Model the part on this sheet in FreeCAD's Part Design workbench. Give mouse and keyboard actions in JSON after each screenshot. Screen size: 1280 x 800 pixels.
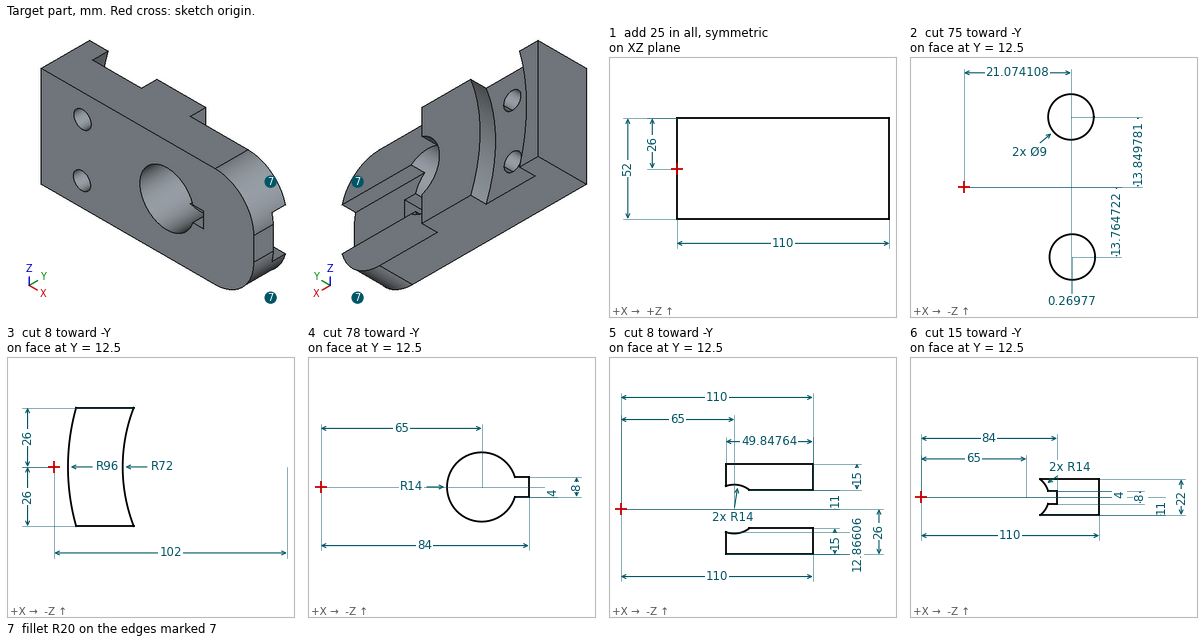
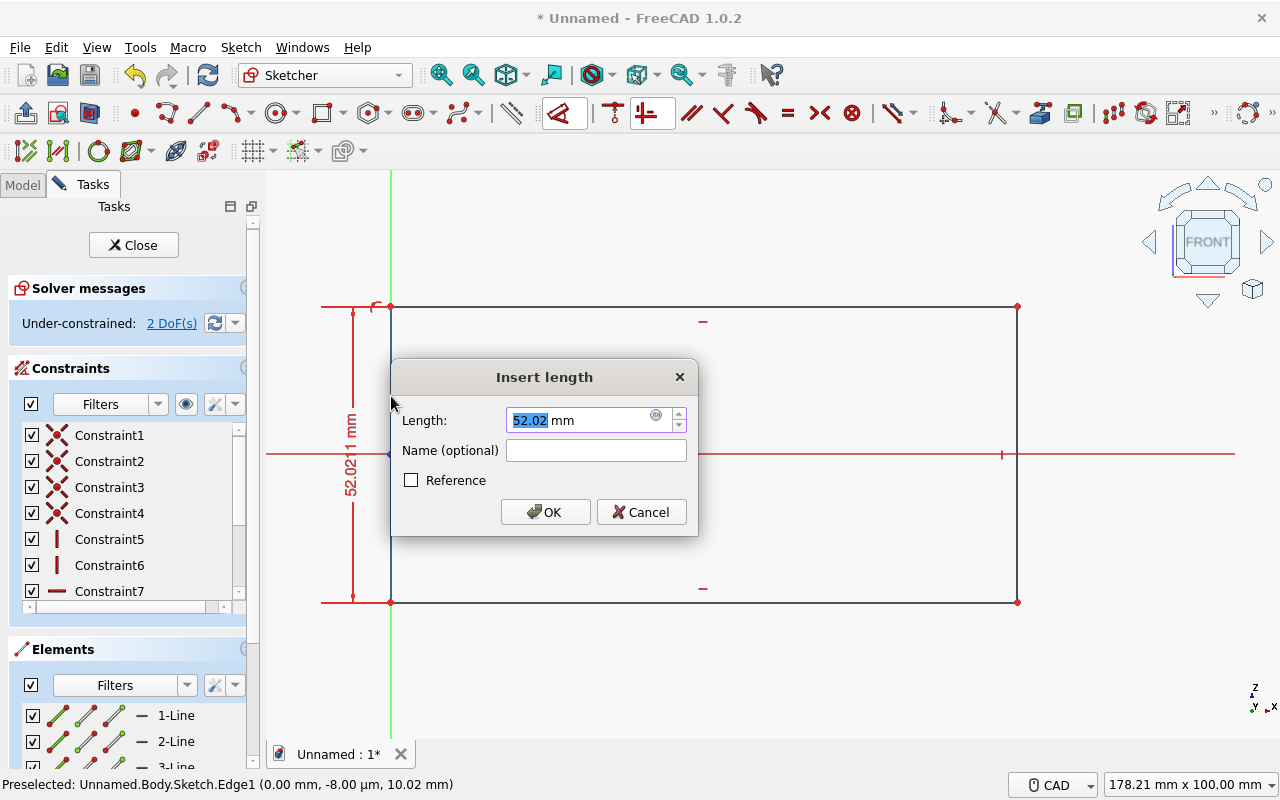
{"action": "type", "text": "52"}
{"action": "key", "text": "Return"}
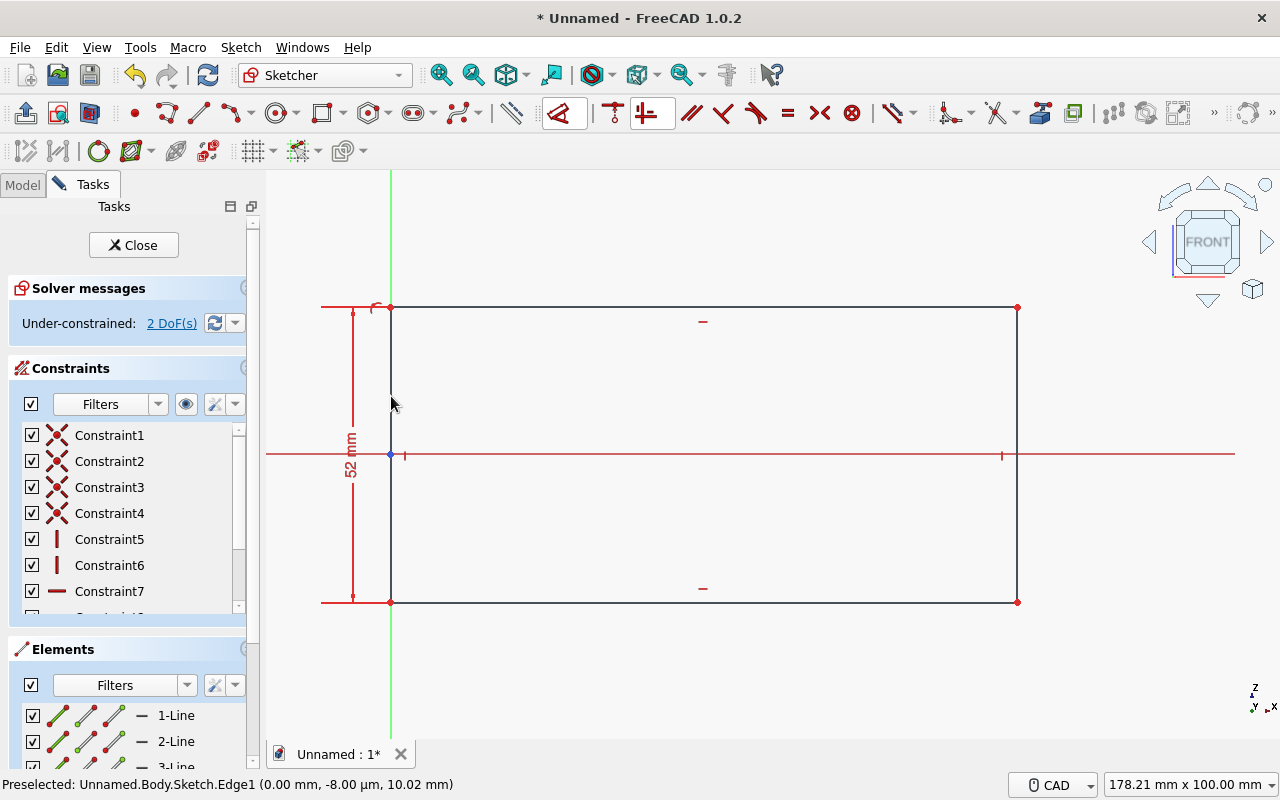
{"action": "left_click", "coordinate": [579, 603]}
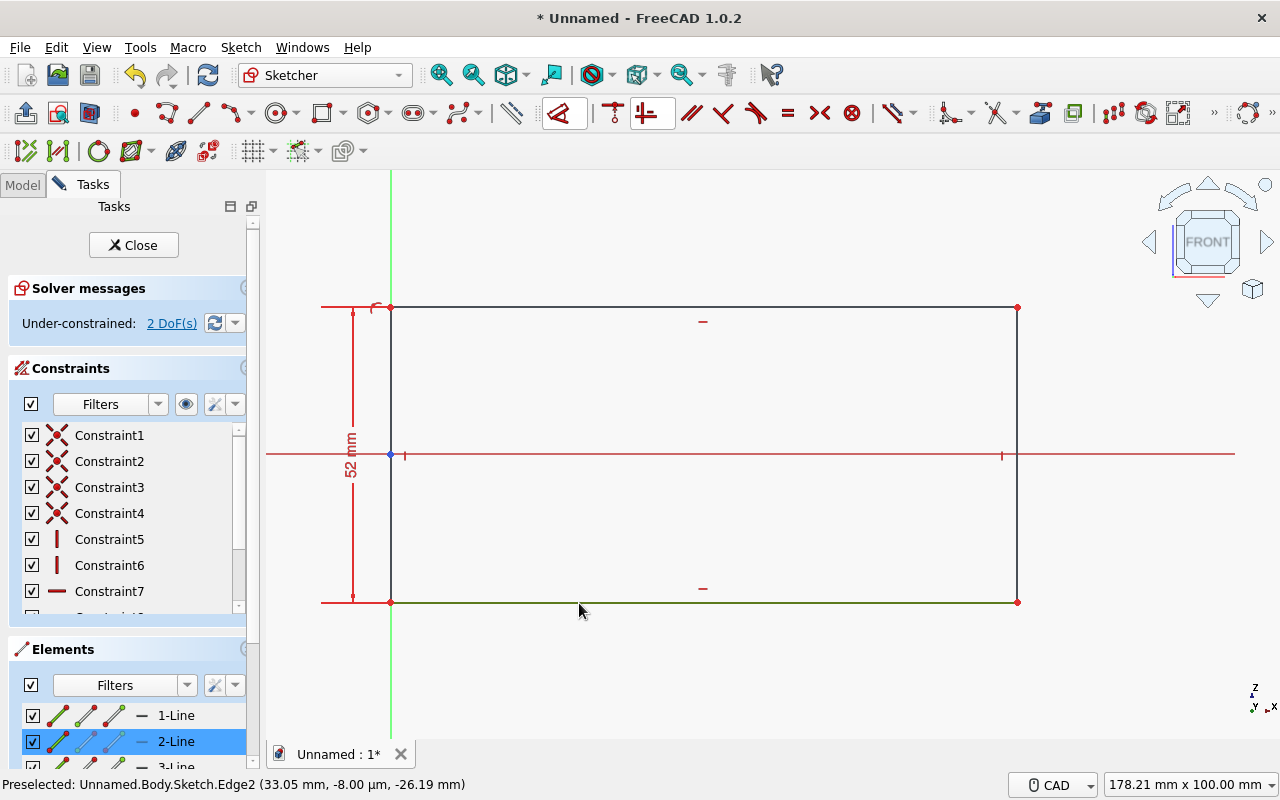
{"action": "left_click", "coordinate": [582, 114]}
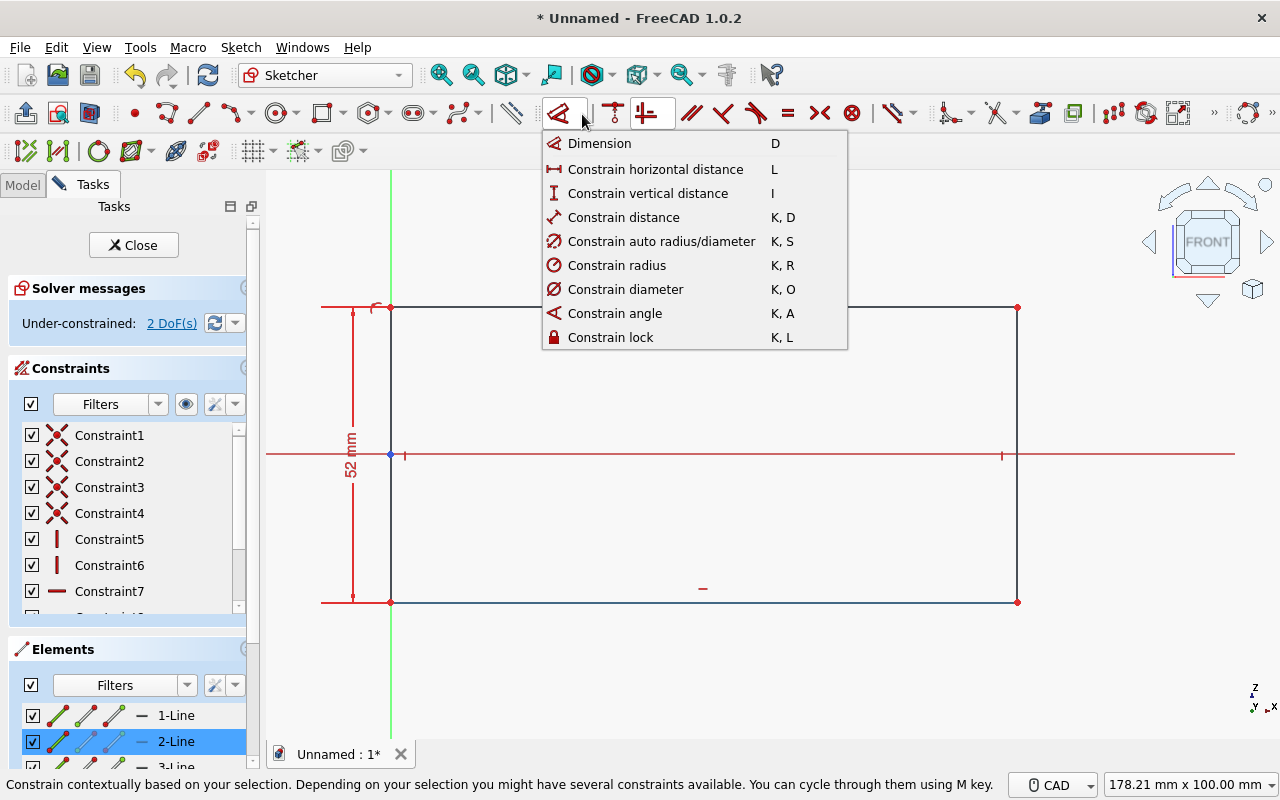
{"action": "left_click", "coordinate": [695, 169]}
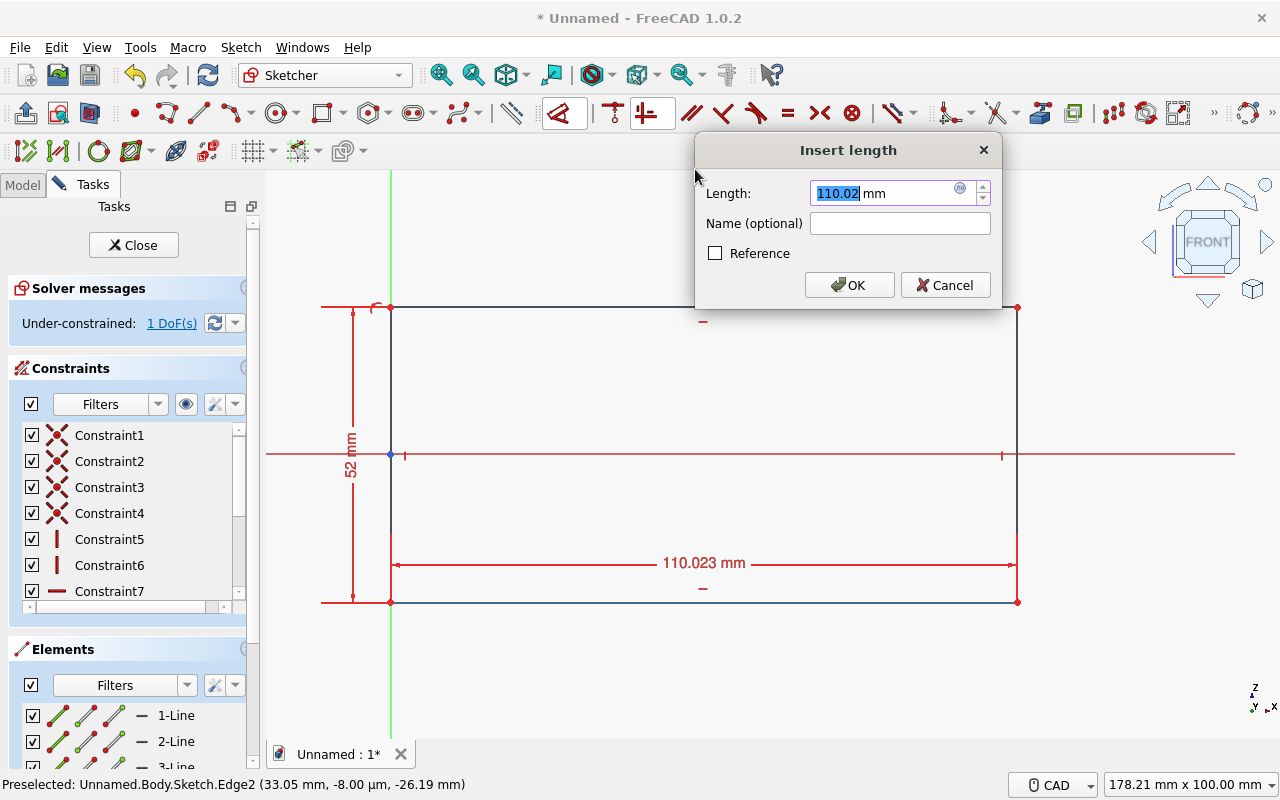
{"action": "type", "text": "110"}
{"action": "key", "text": "Return"}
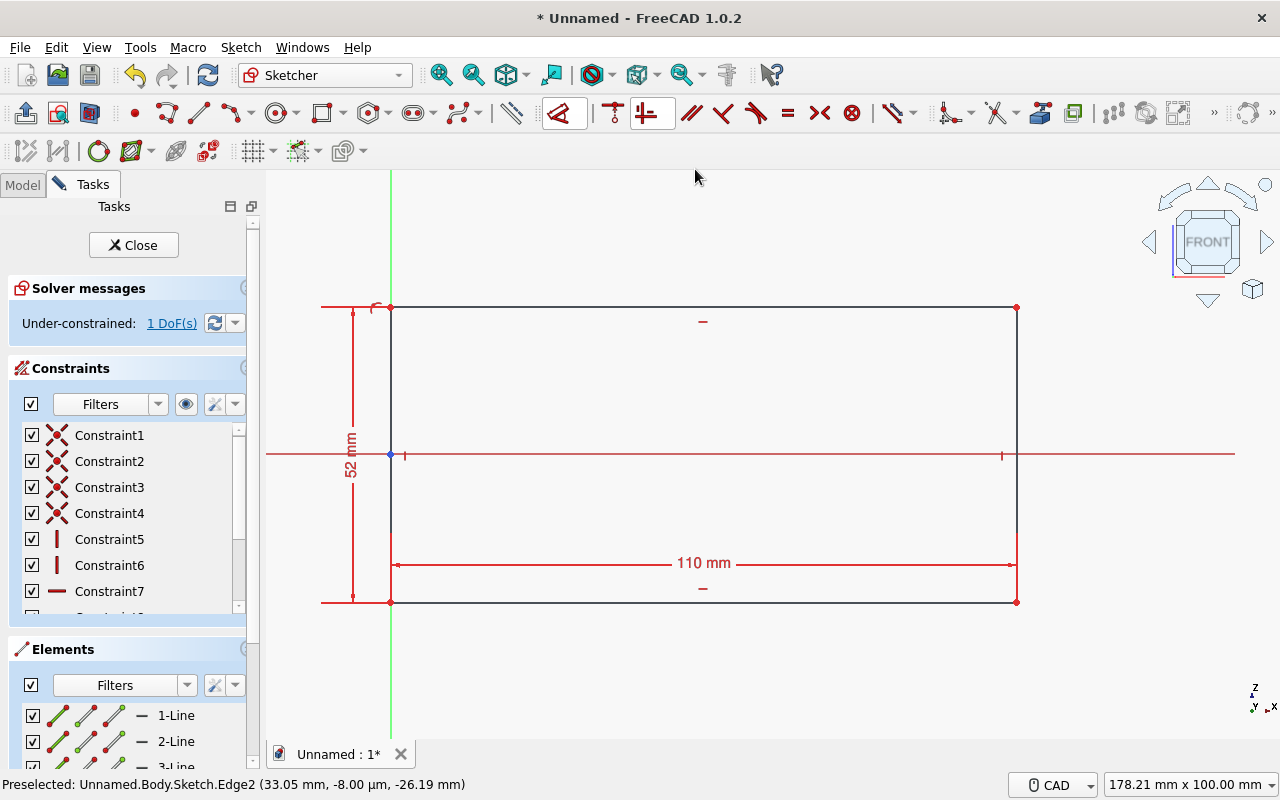
{"action": "left_click", "coordinate": [391, 307]}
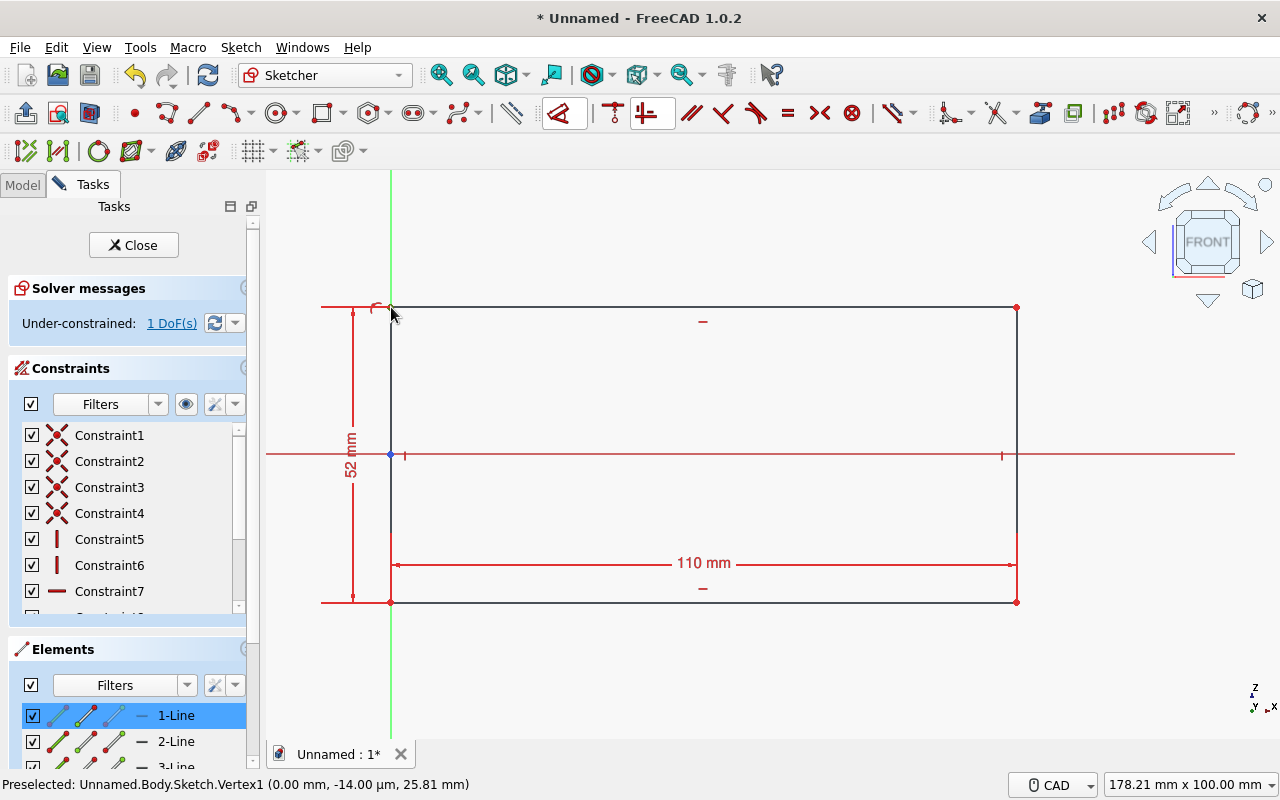
{"action": "left_click", "coordinate": [582, 114]}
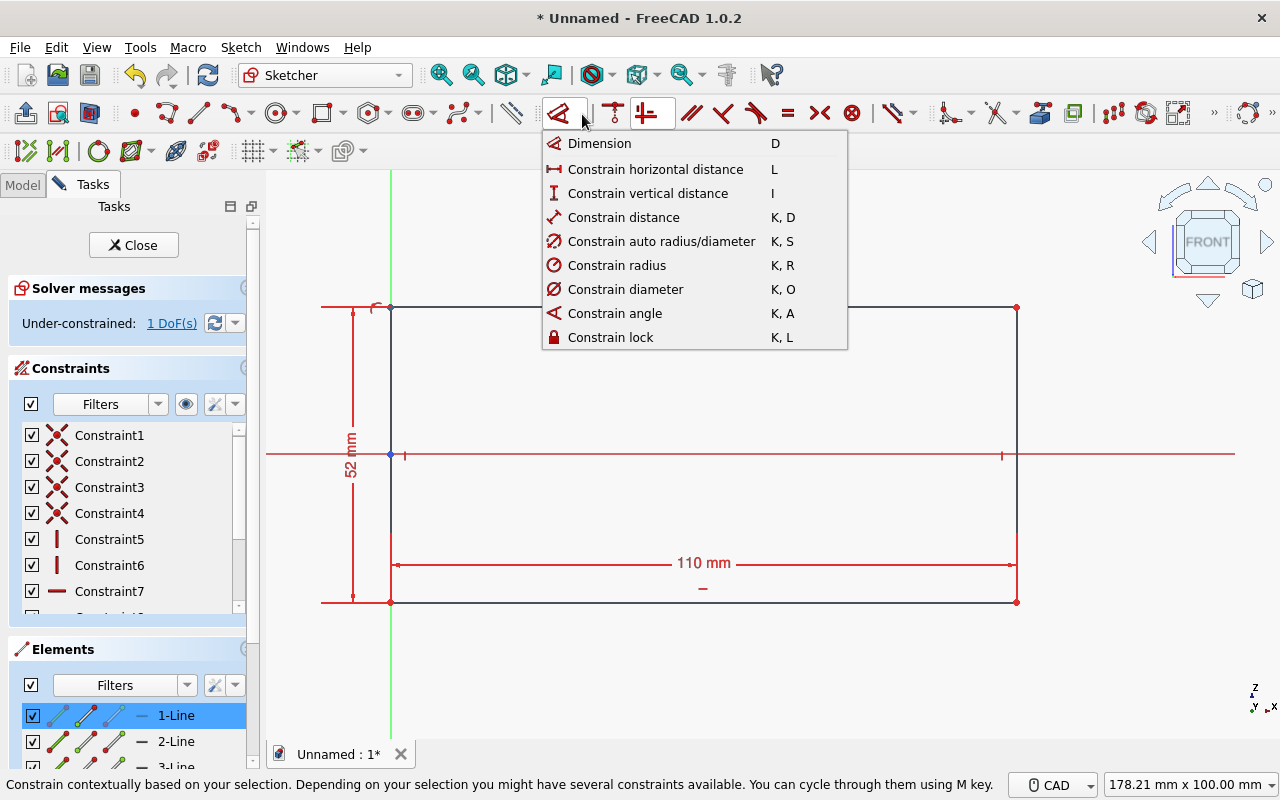
{"action": "left_click", "coordinate": [695, 193]}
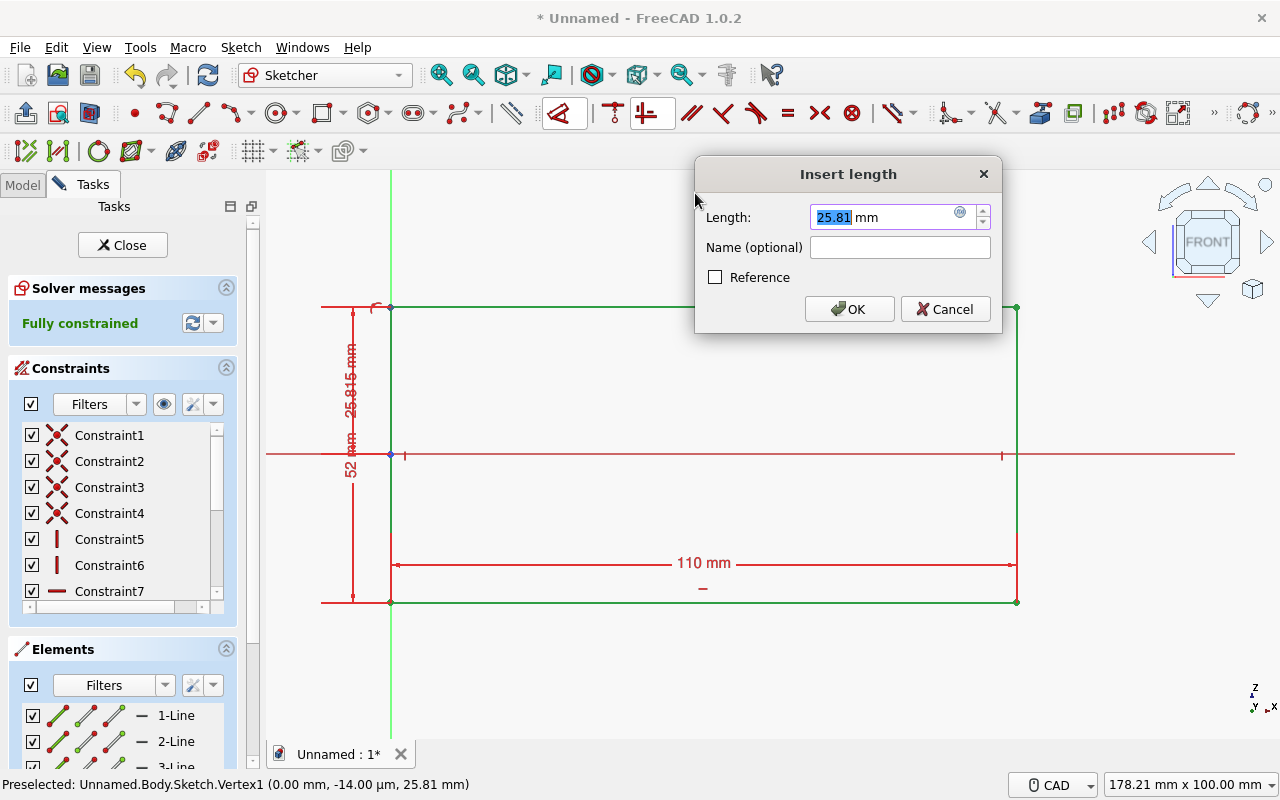
{"action": "type", "text": "26"}
{"action": "key", "text": "Return"}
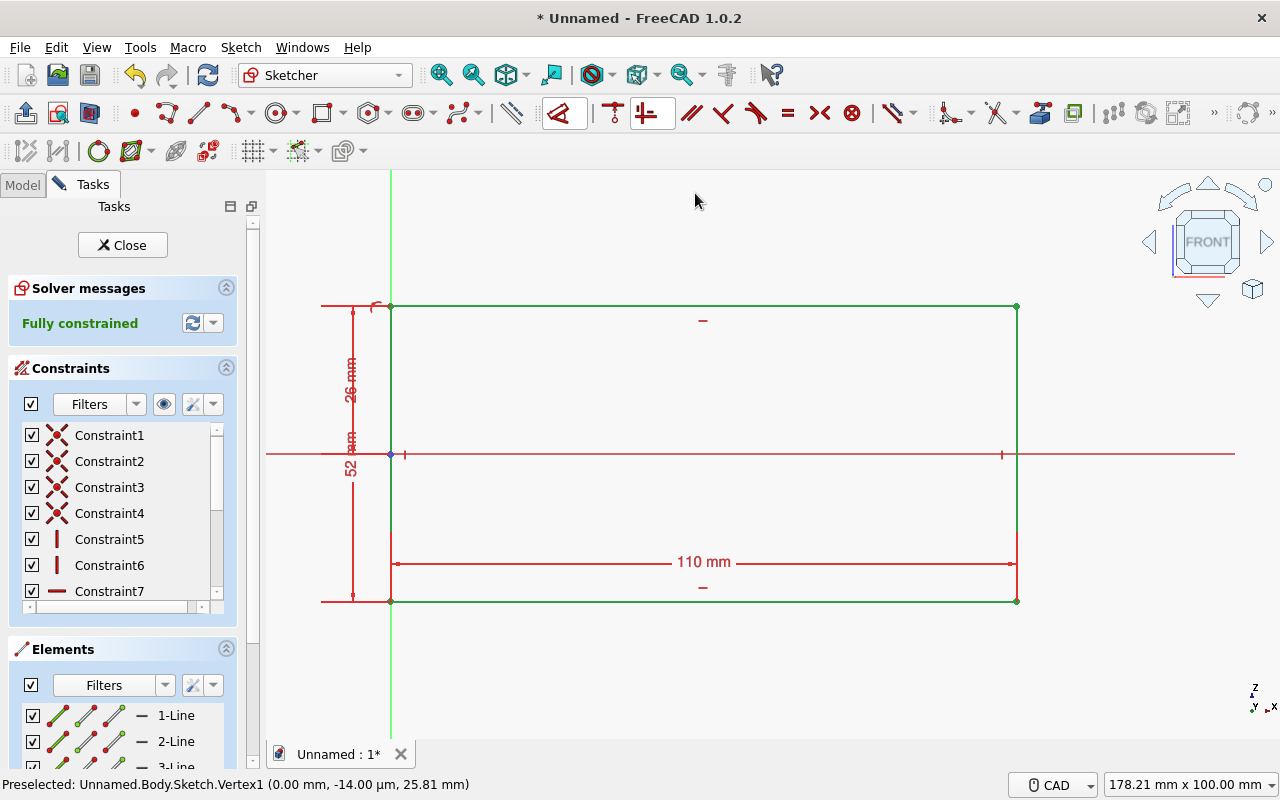
{"action": "left_click", "coordinate": [123, 245]}